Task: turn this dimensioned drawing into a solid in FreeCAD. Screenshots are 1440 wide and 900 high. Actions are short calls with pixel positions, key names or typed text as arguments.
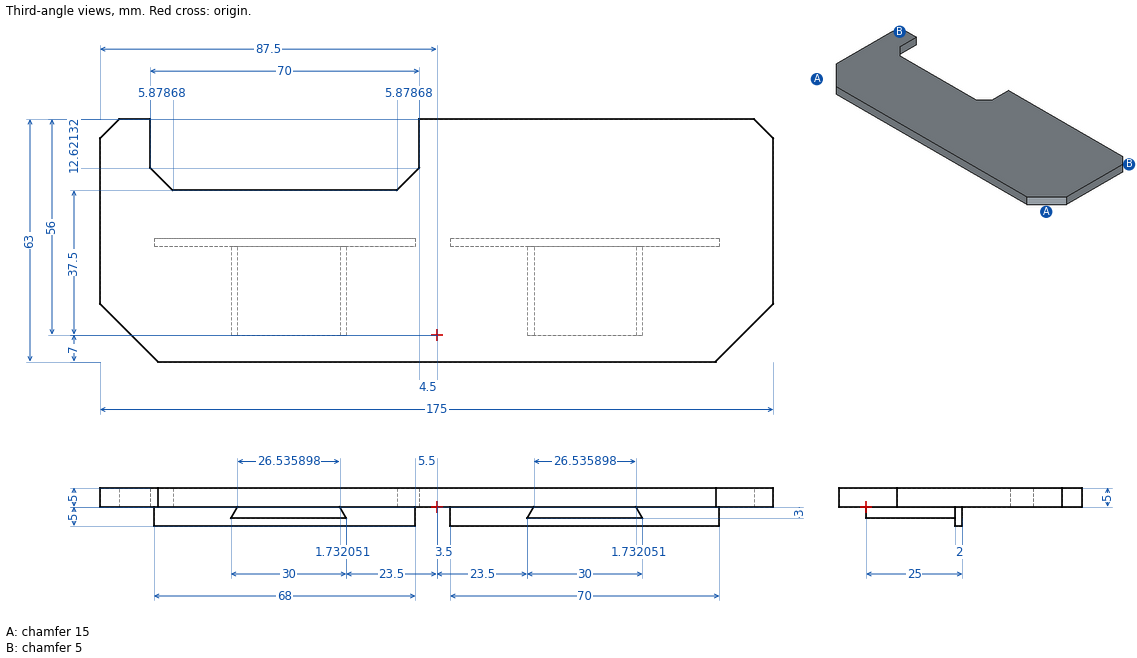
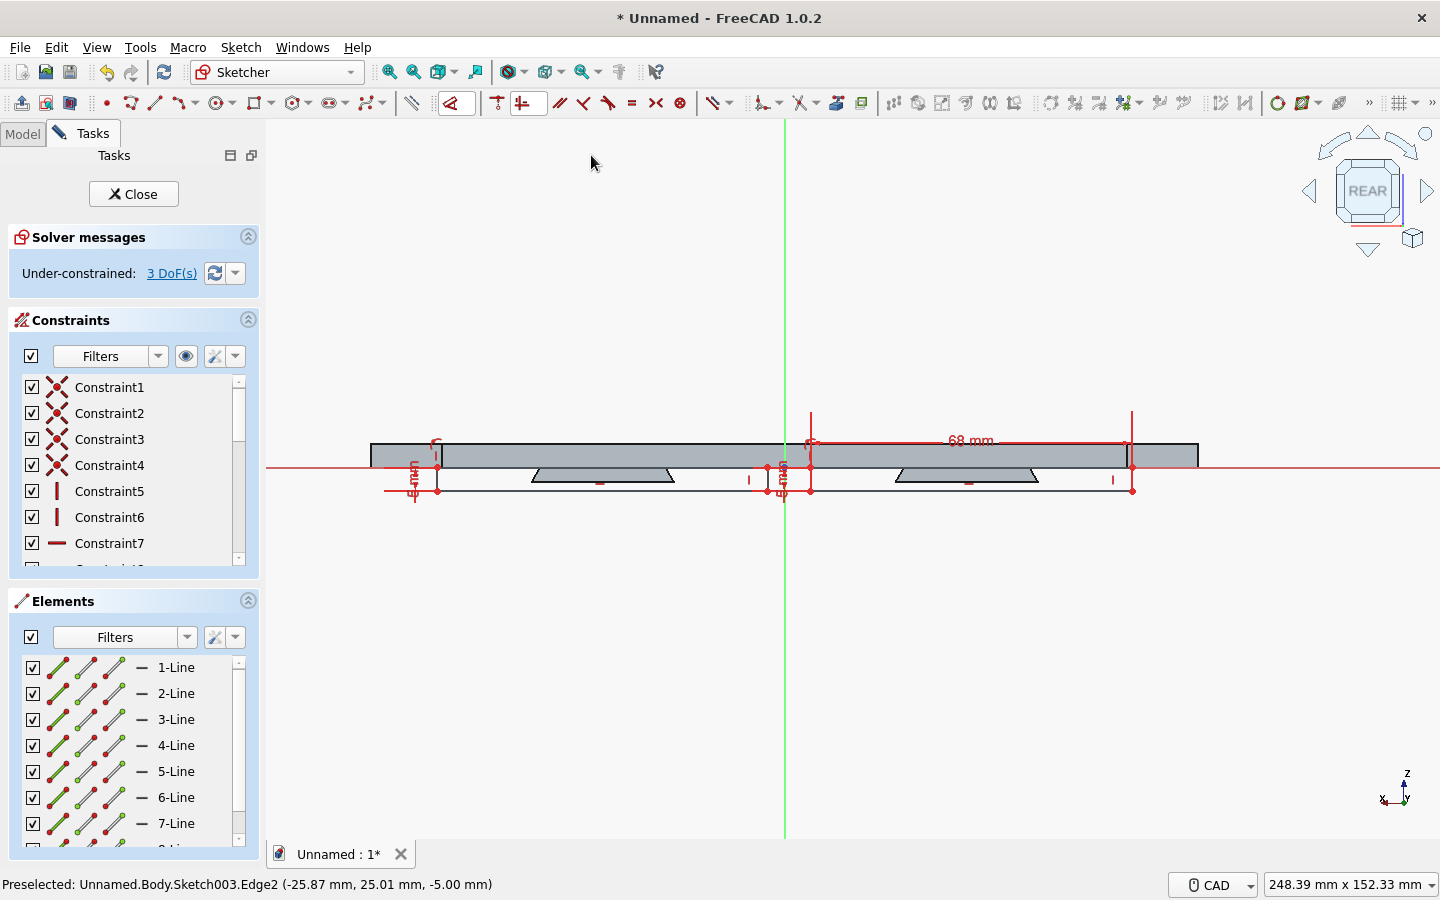
click(536, 491)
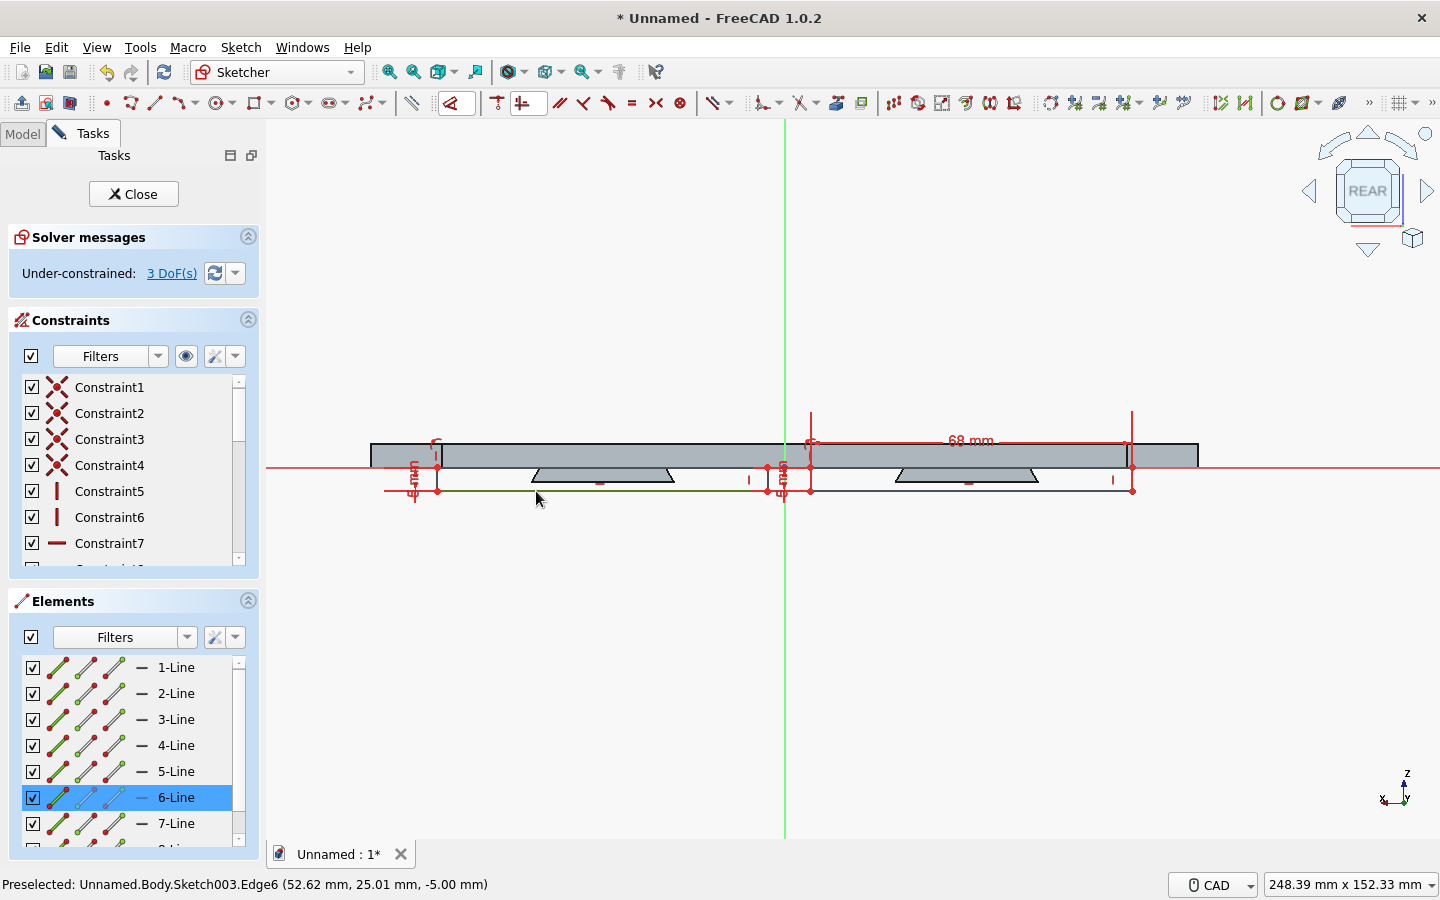
click(470, 104)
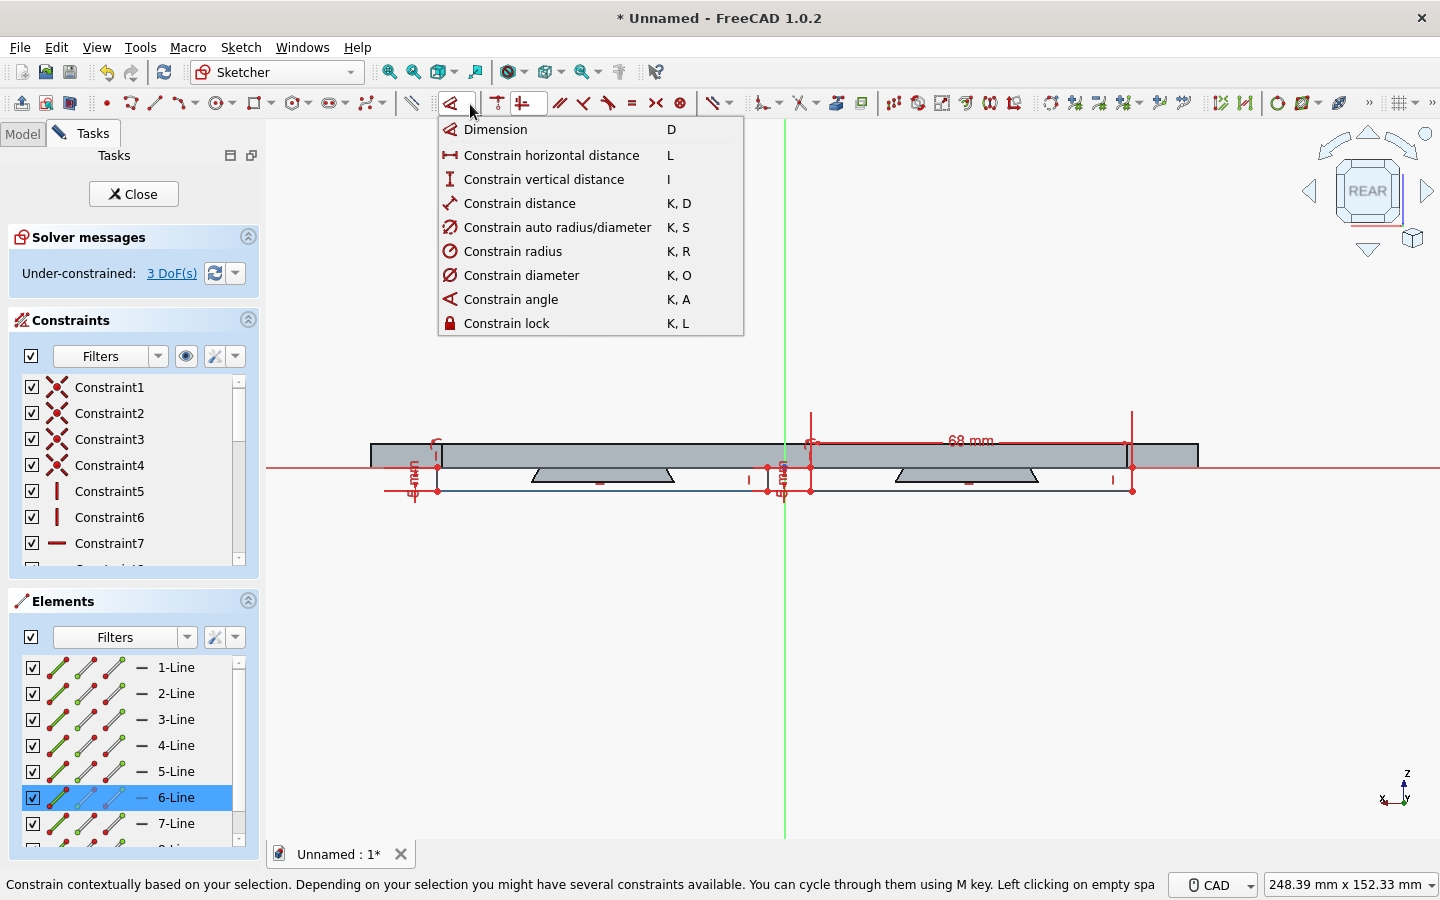
click(591, 155)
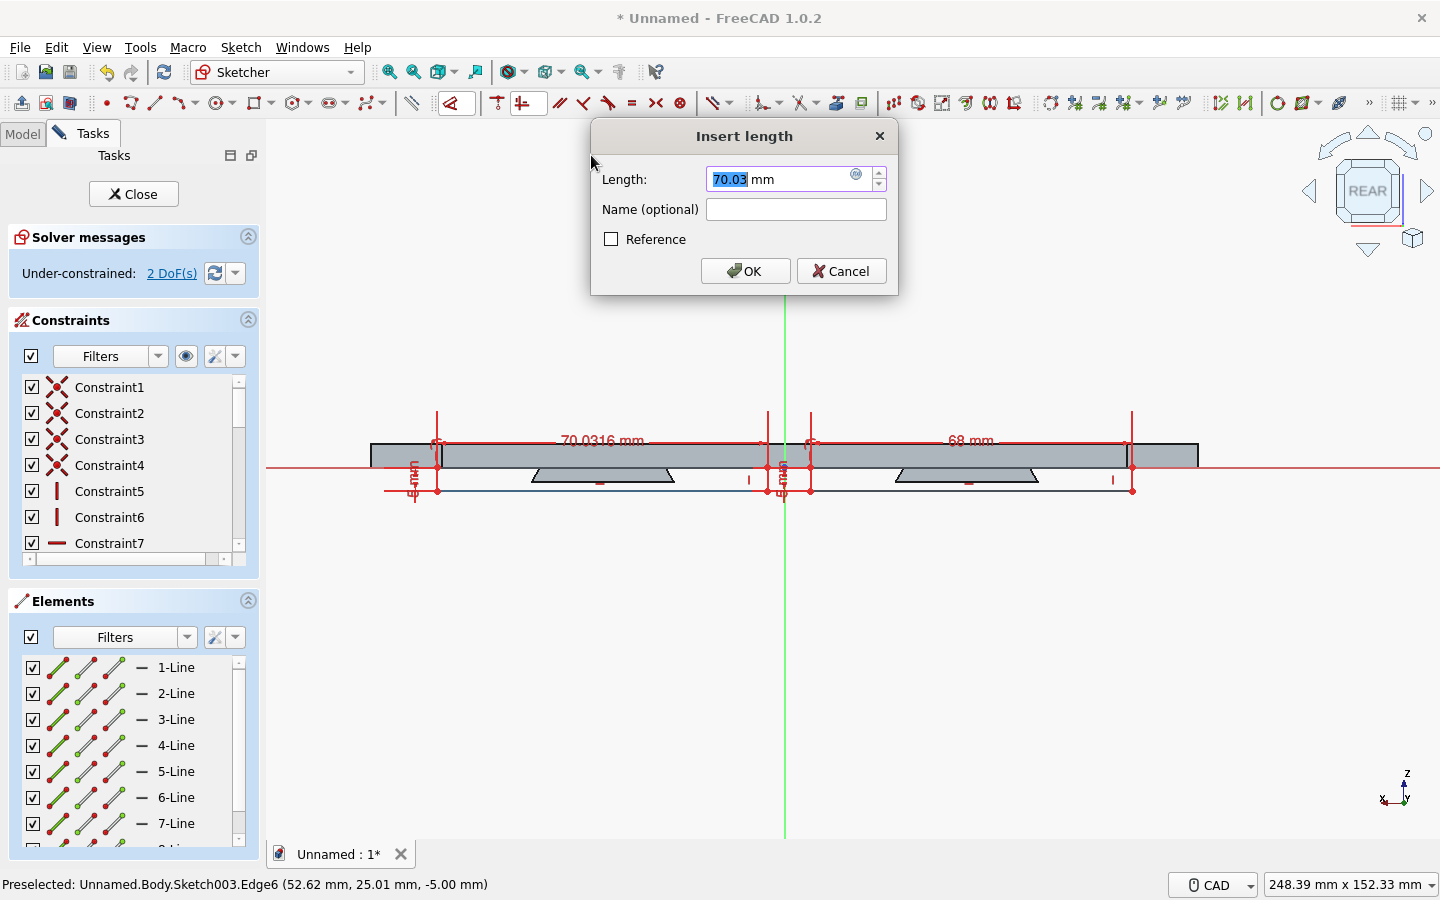
text(70)
key(Return)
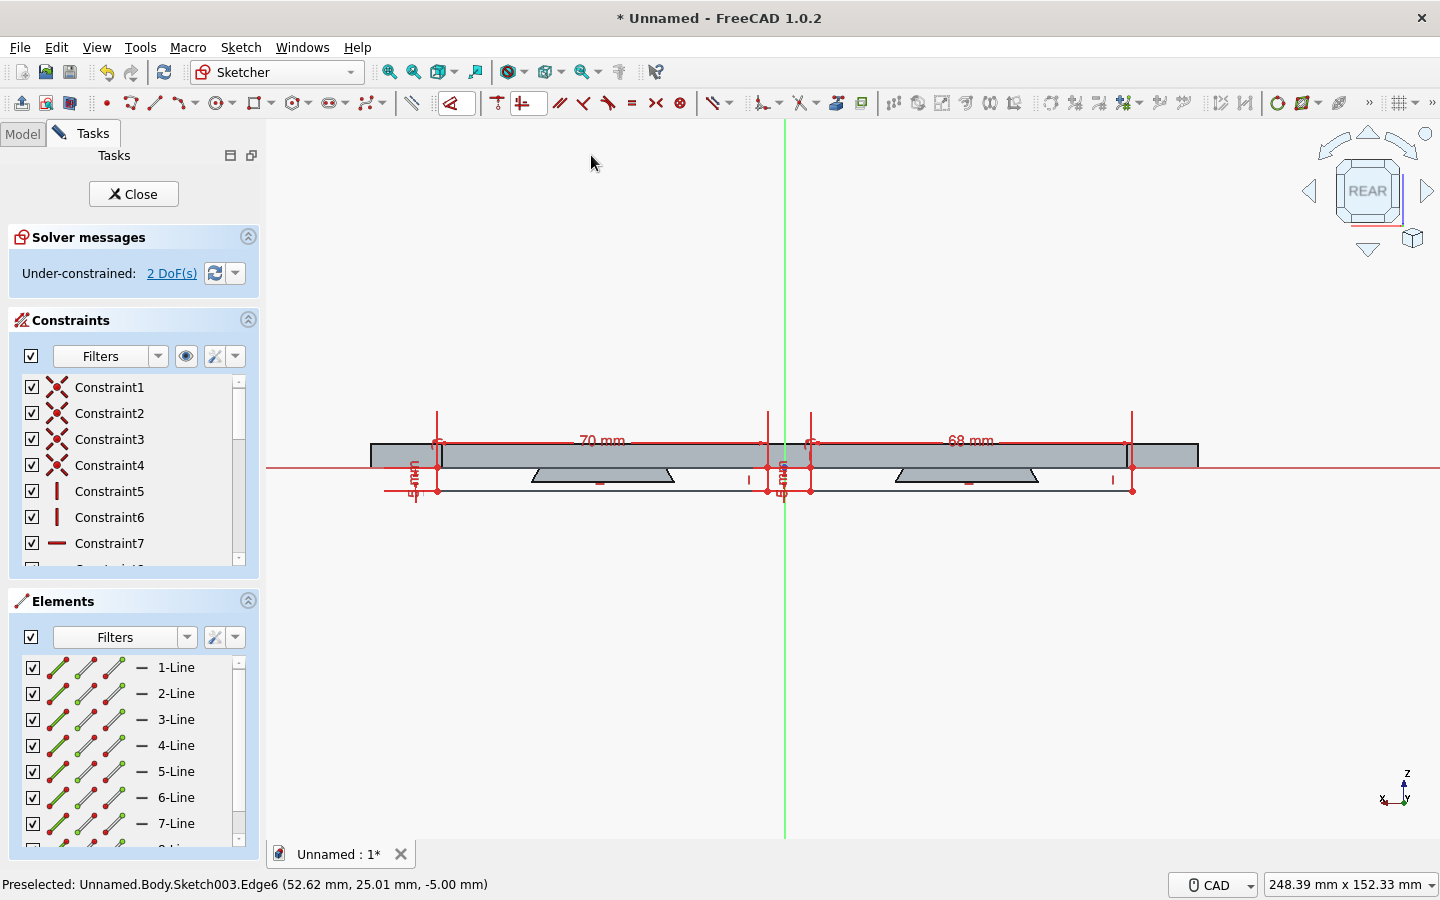
scroll(811, 468, up, 3)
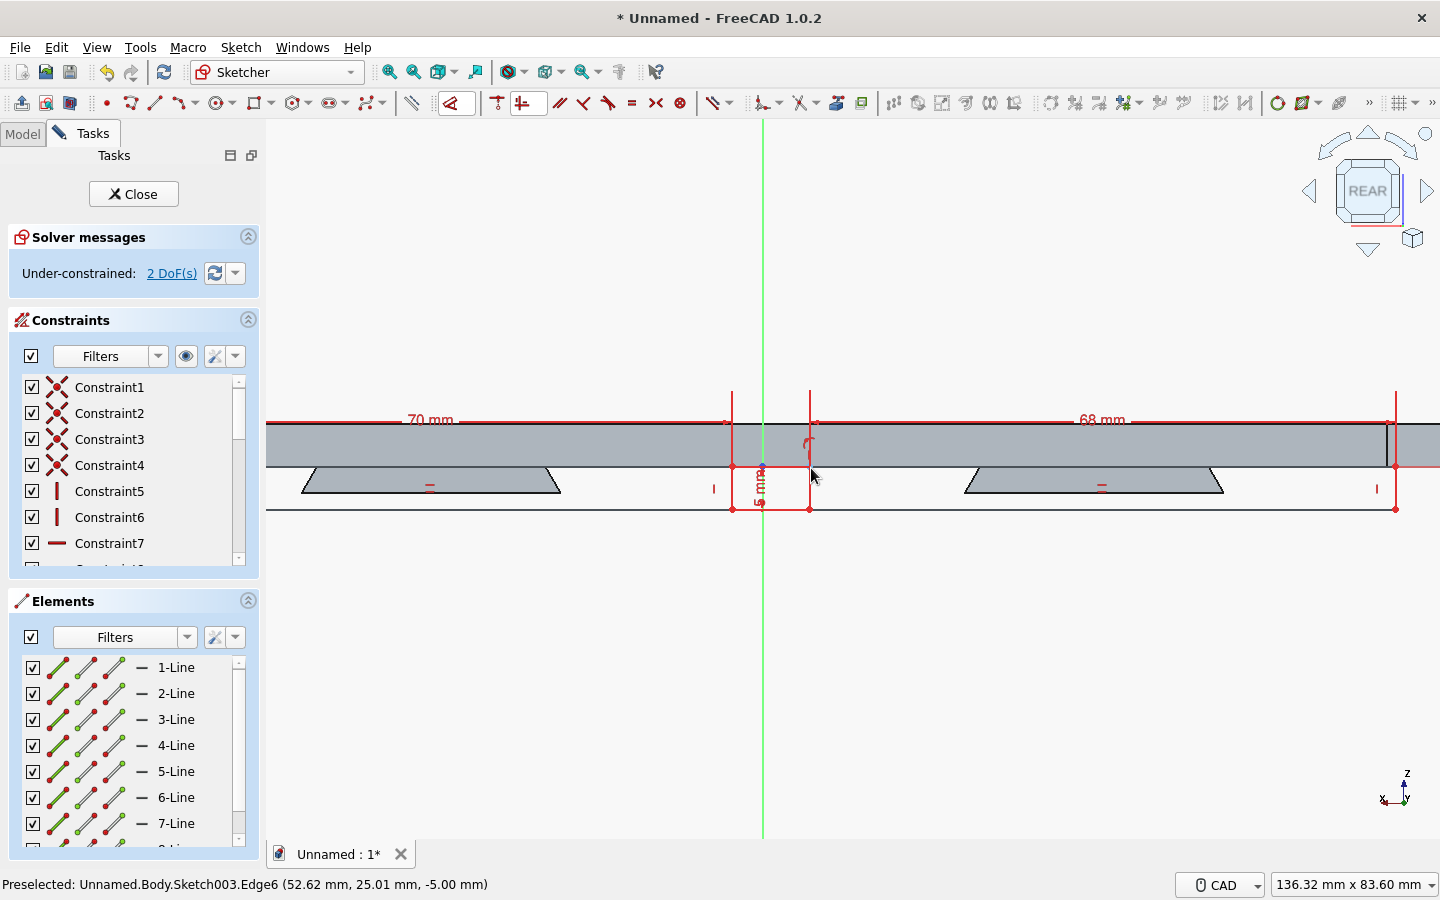
click(810, 467)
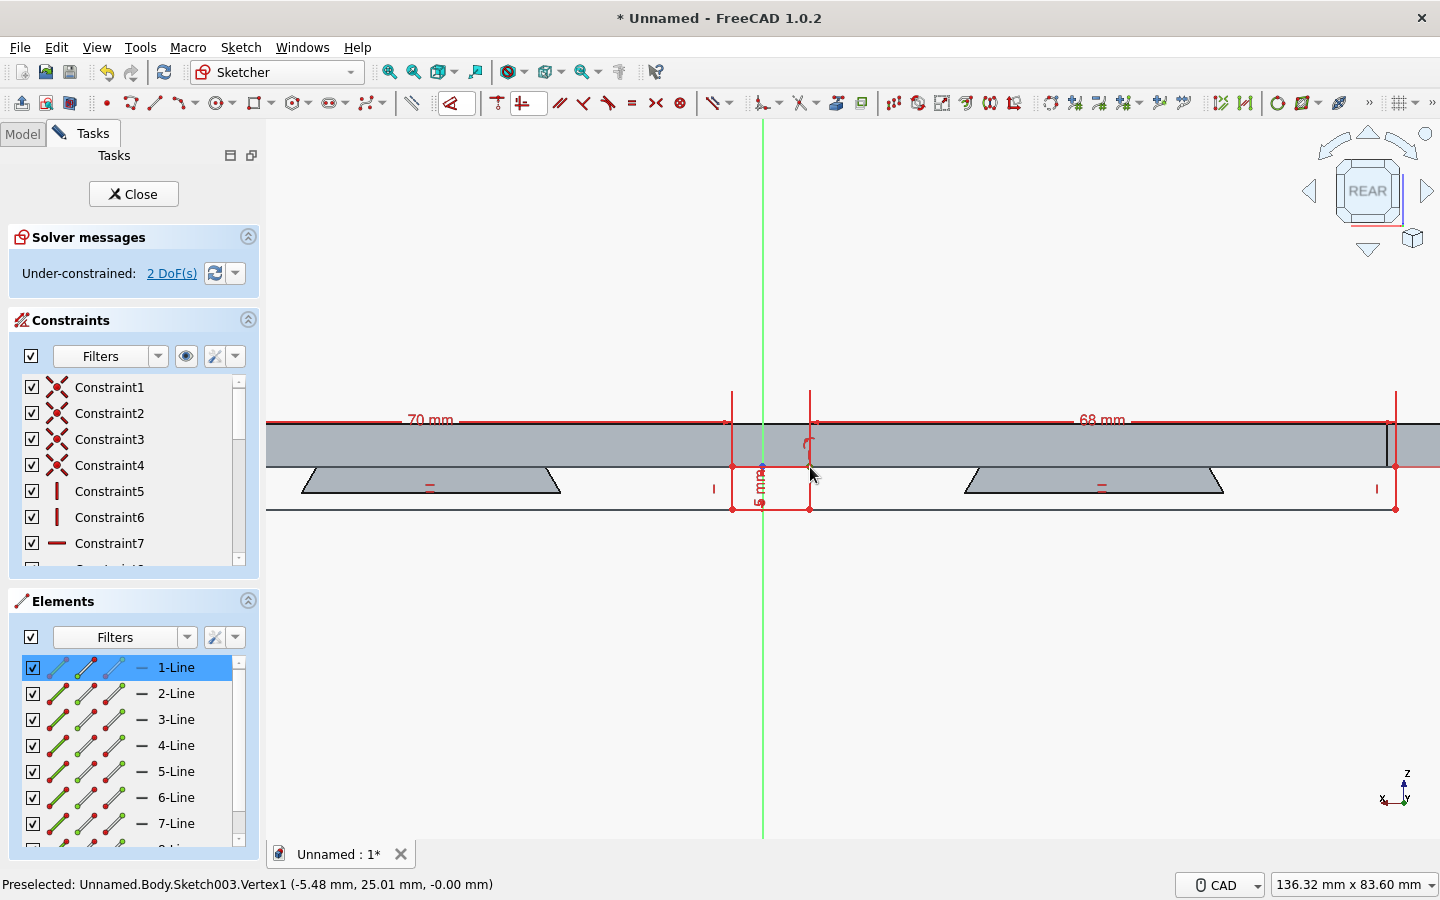
key(l)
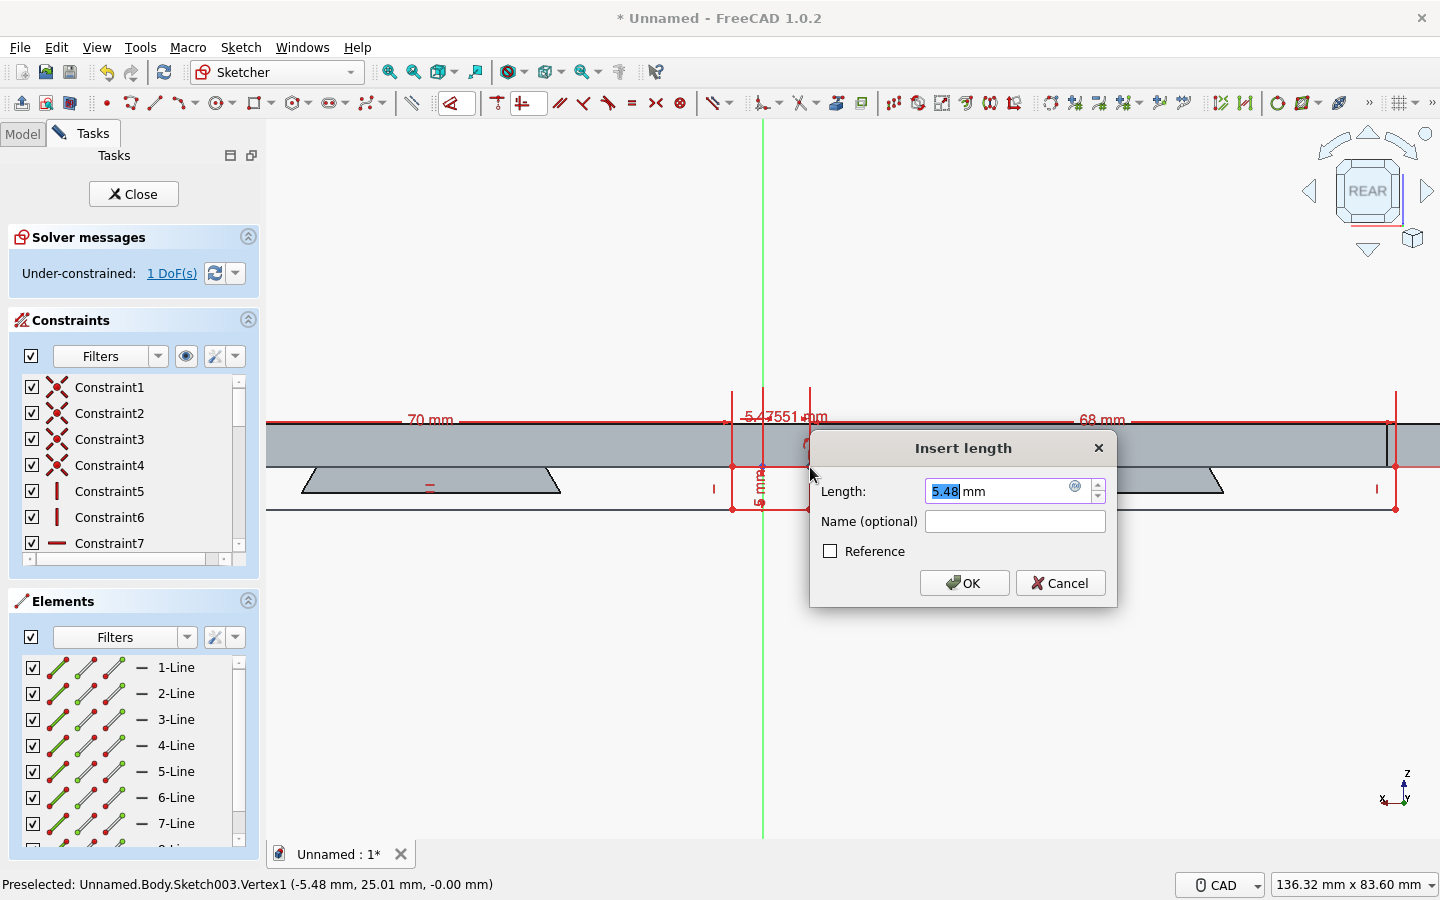
text(5.5)
key(Return)